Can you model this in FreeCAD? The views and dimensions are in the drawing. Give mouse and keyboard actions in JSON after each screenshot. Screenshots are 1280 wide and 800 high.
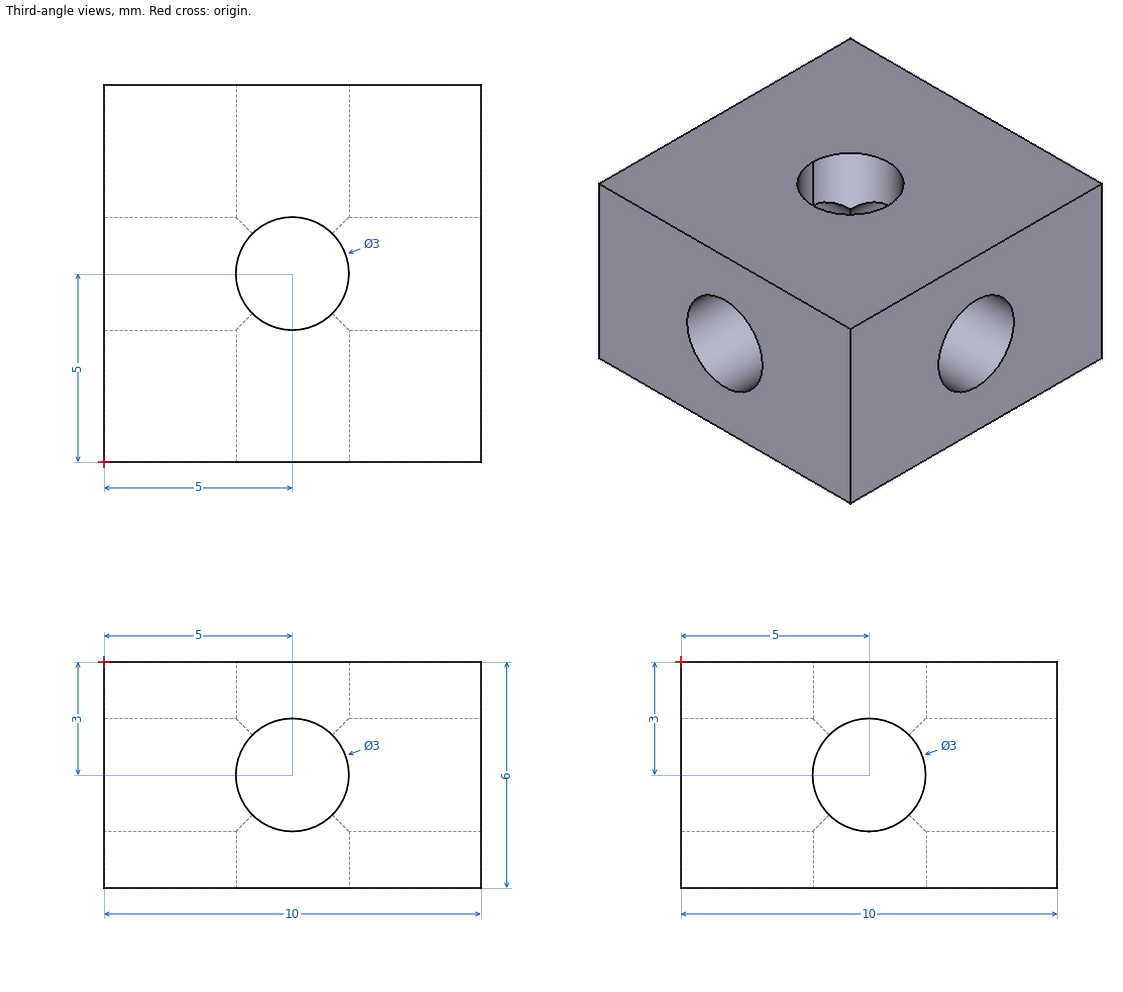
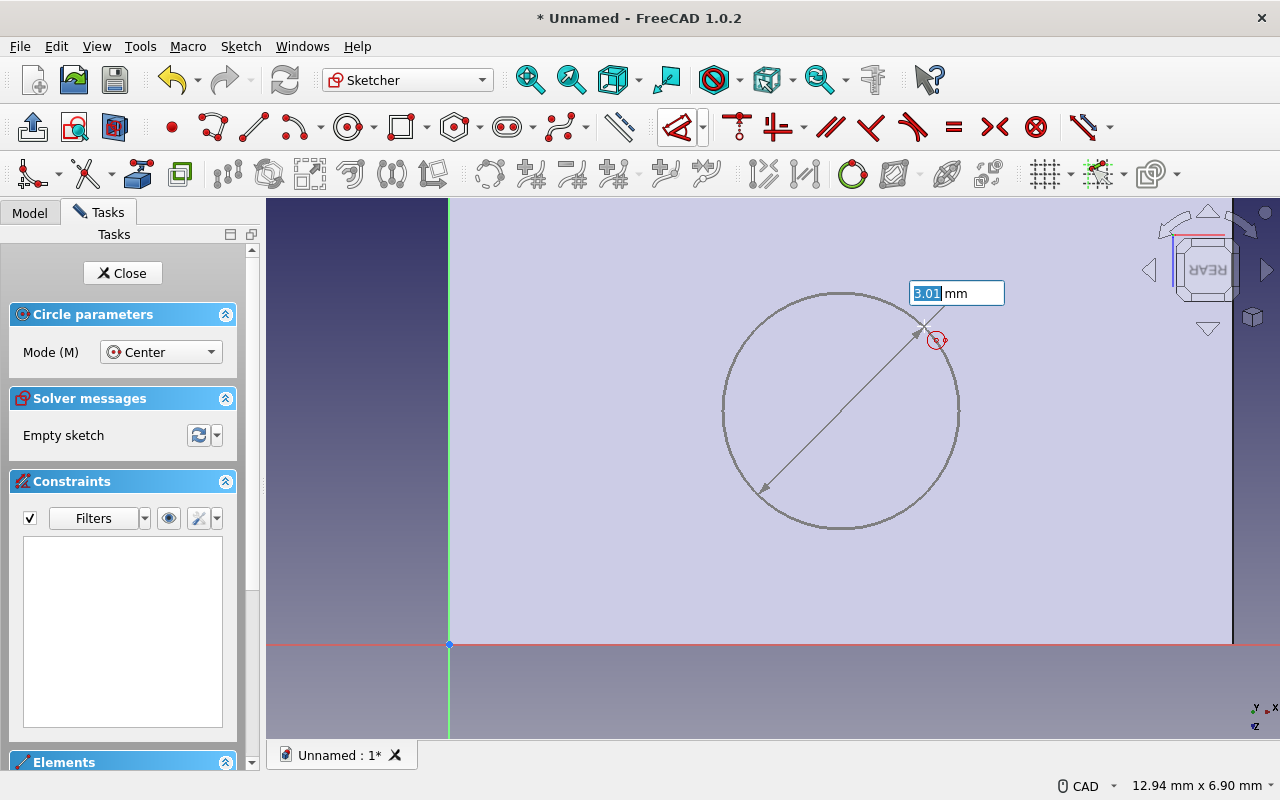
{"action": "type", "text": "3"}
{"action": "key", "text": "Return"}
{"action": "key", "text": "Escape"}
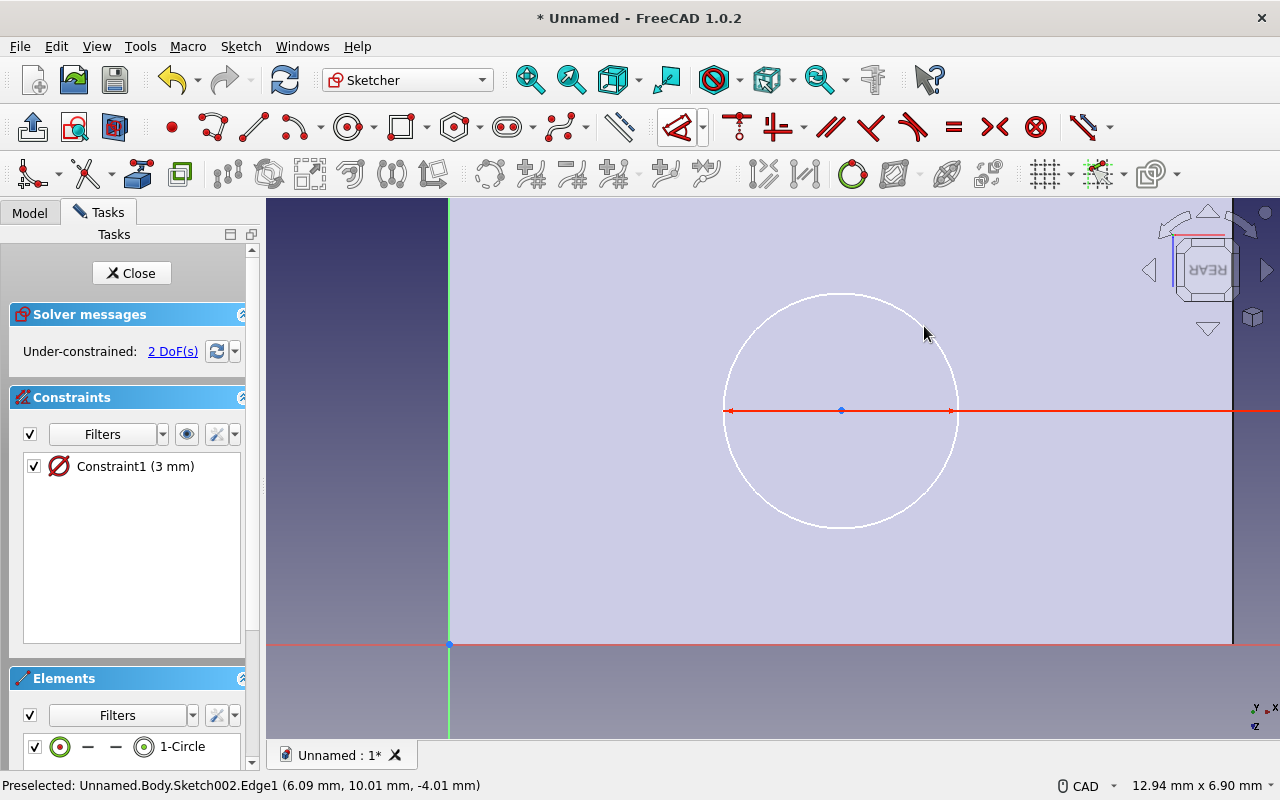
{"action": "left_click", "coordinate": [841, 411]}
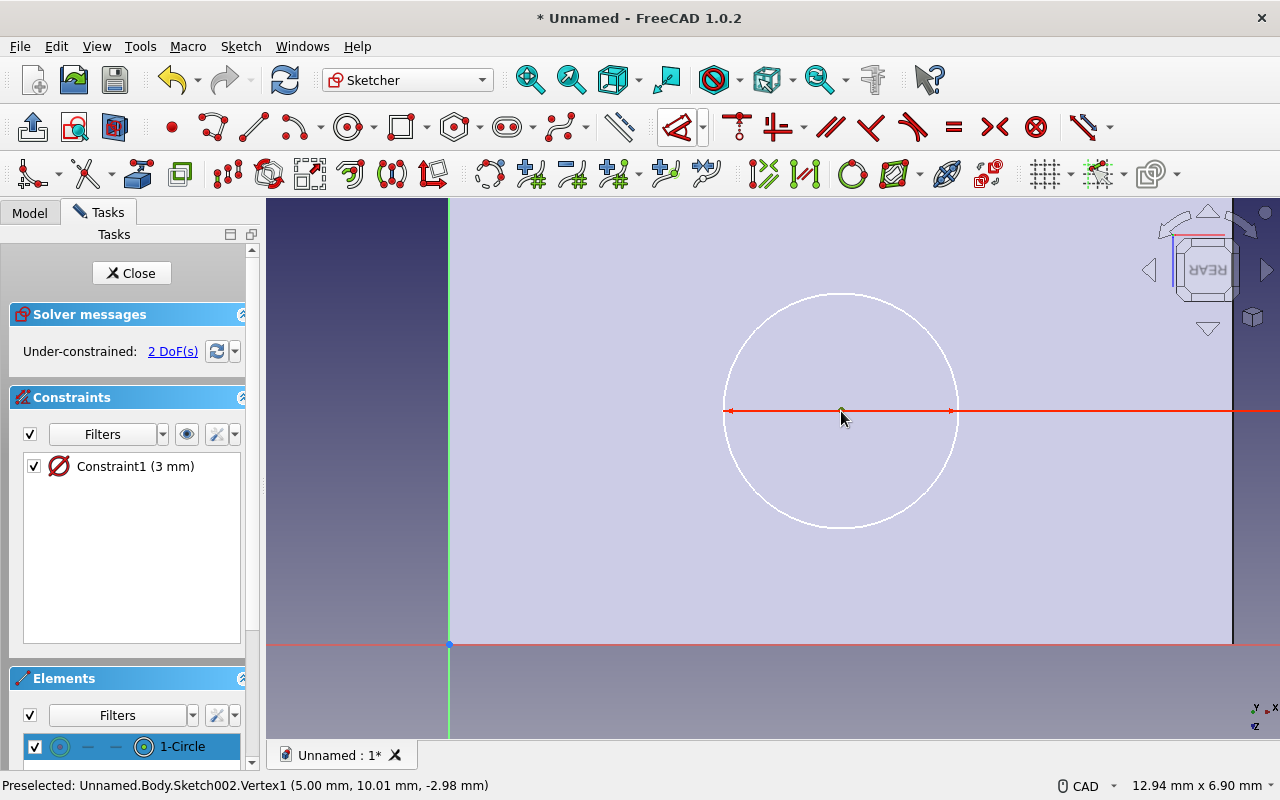
{"action": "key", "text": "l"}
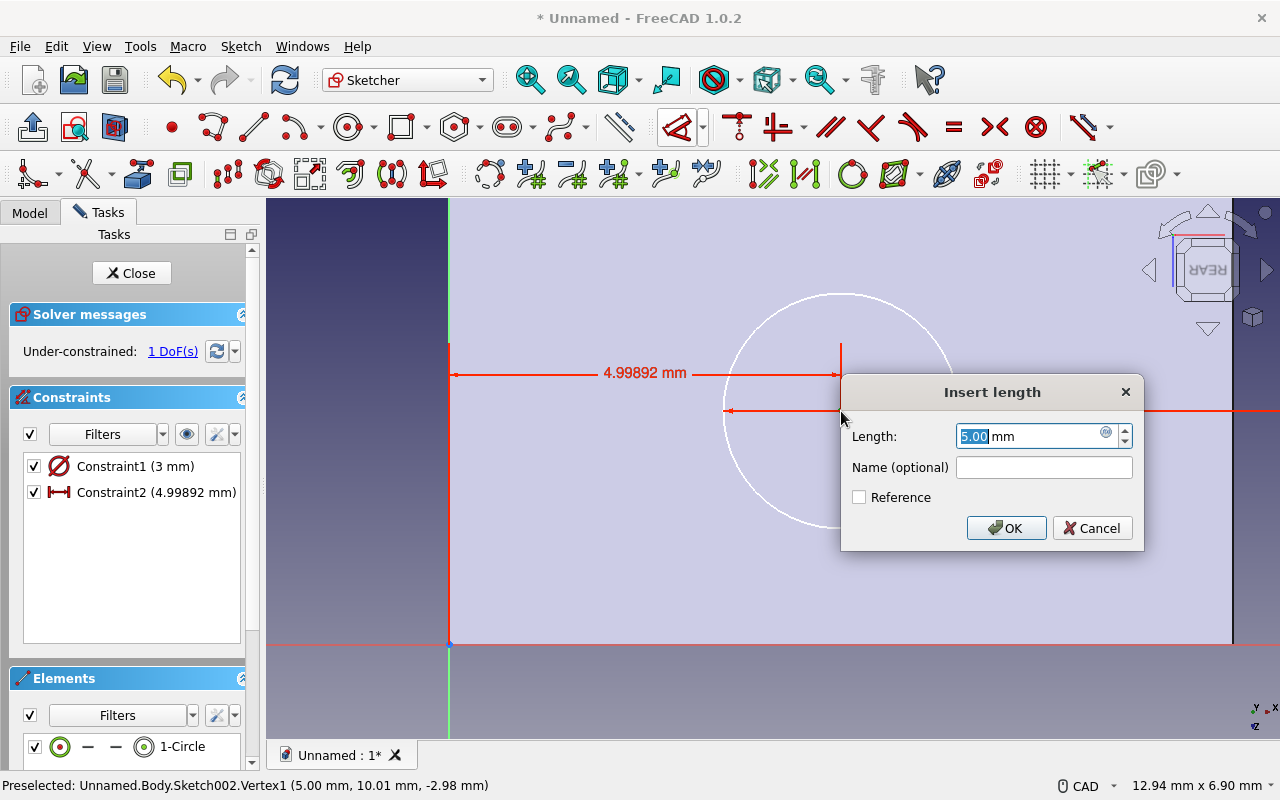
{"action": "type", "text": "5"}
{"action": "key", "text": "Return"}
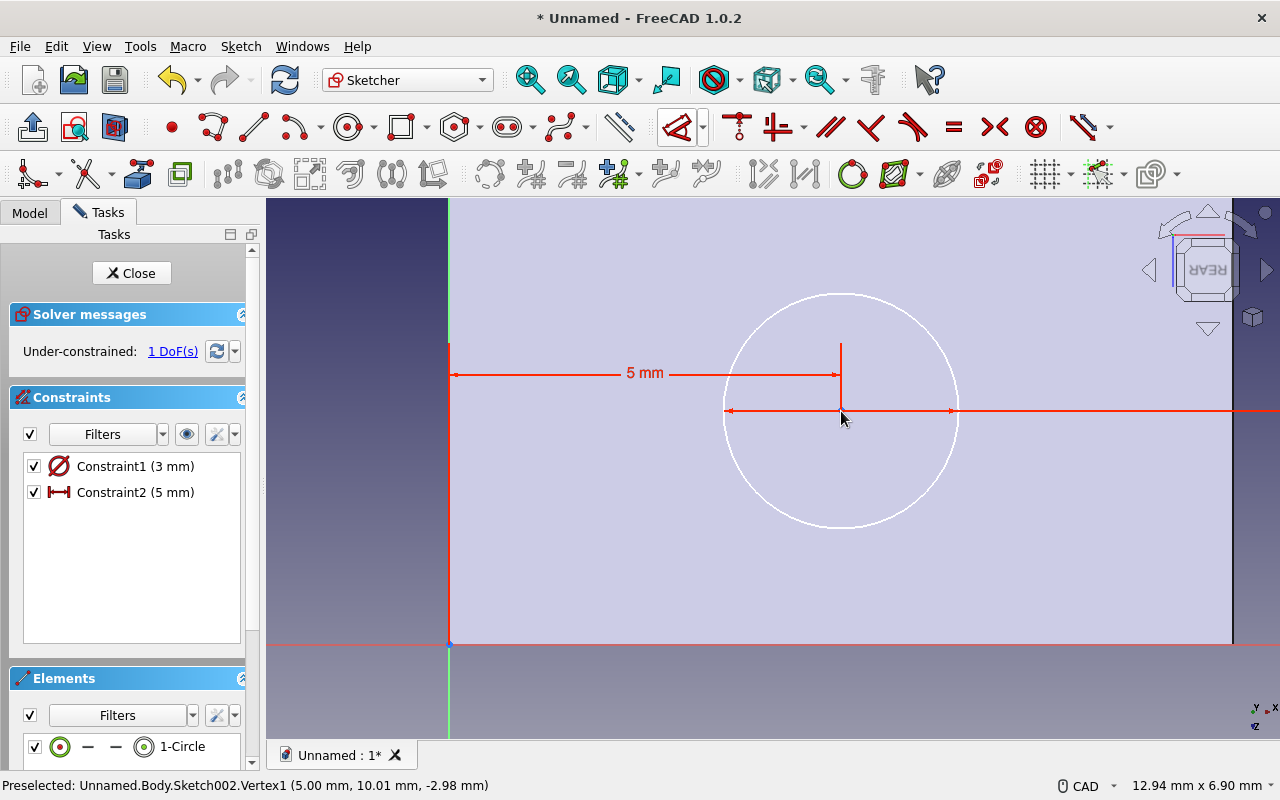
{"action": "left_click", "coordinate": [841, 411]}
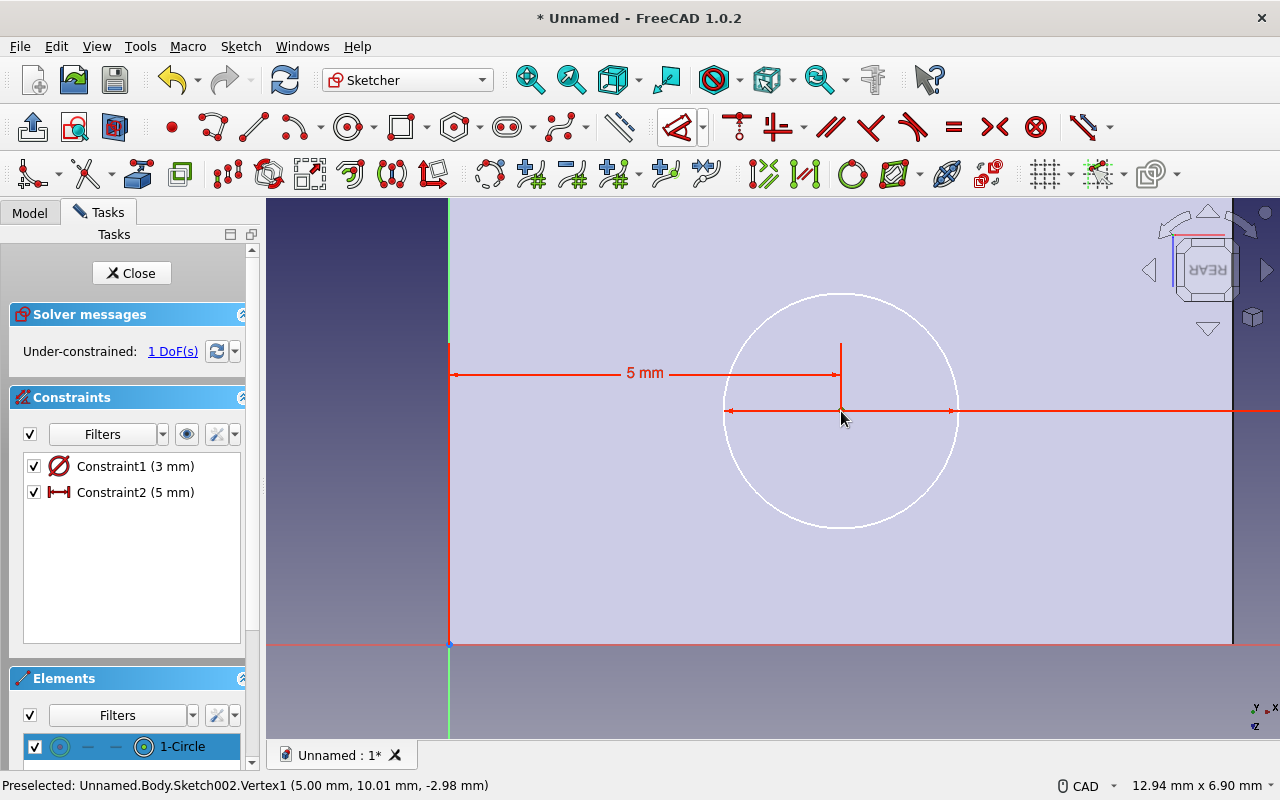
{"action": "left_click", "coordinate": [702, 128]}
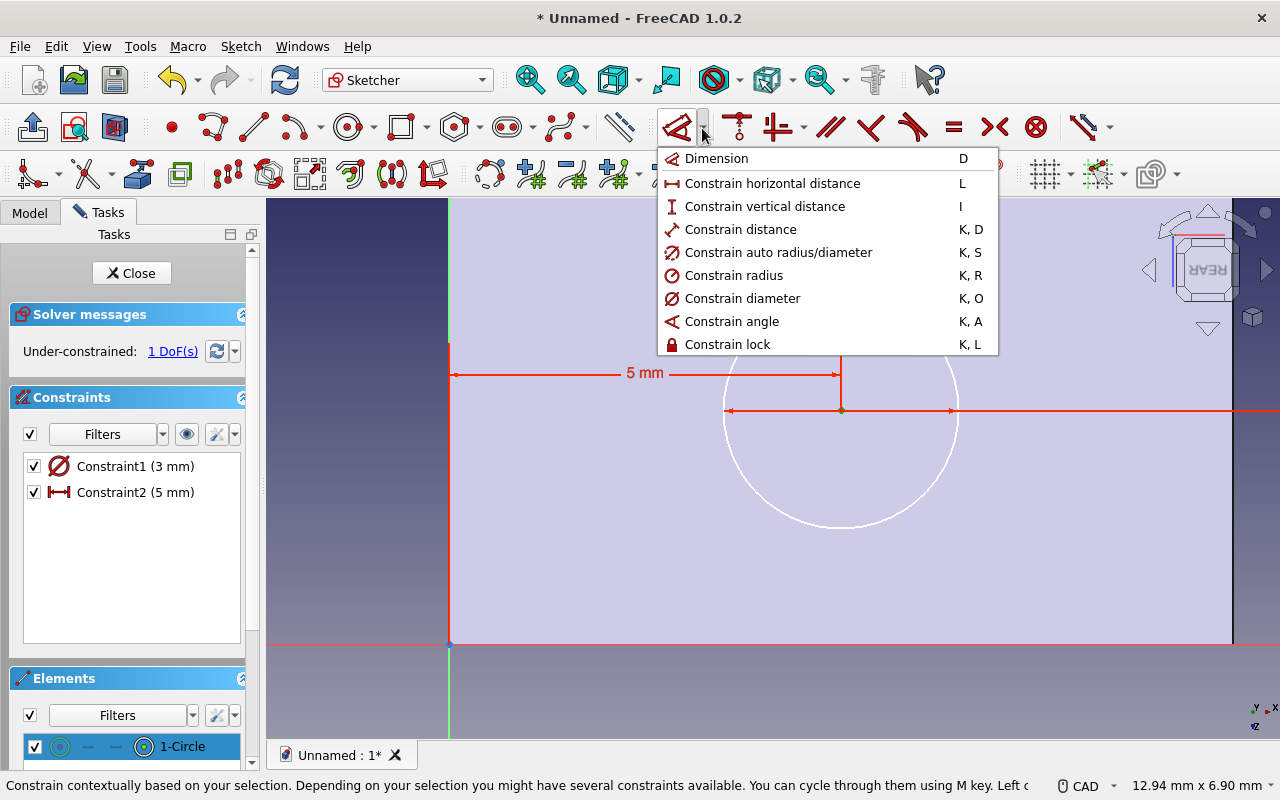
{"action": "left_click", "coordinate": [828, 206]}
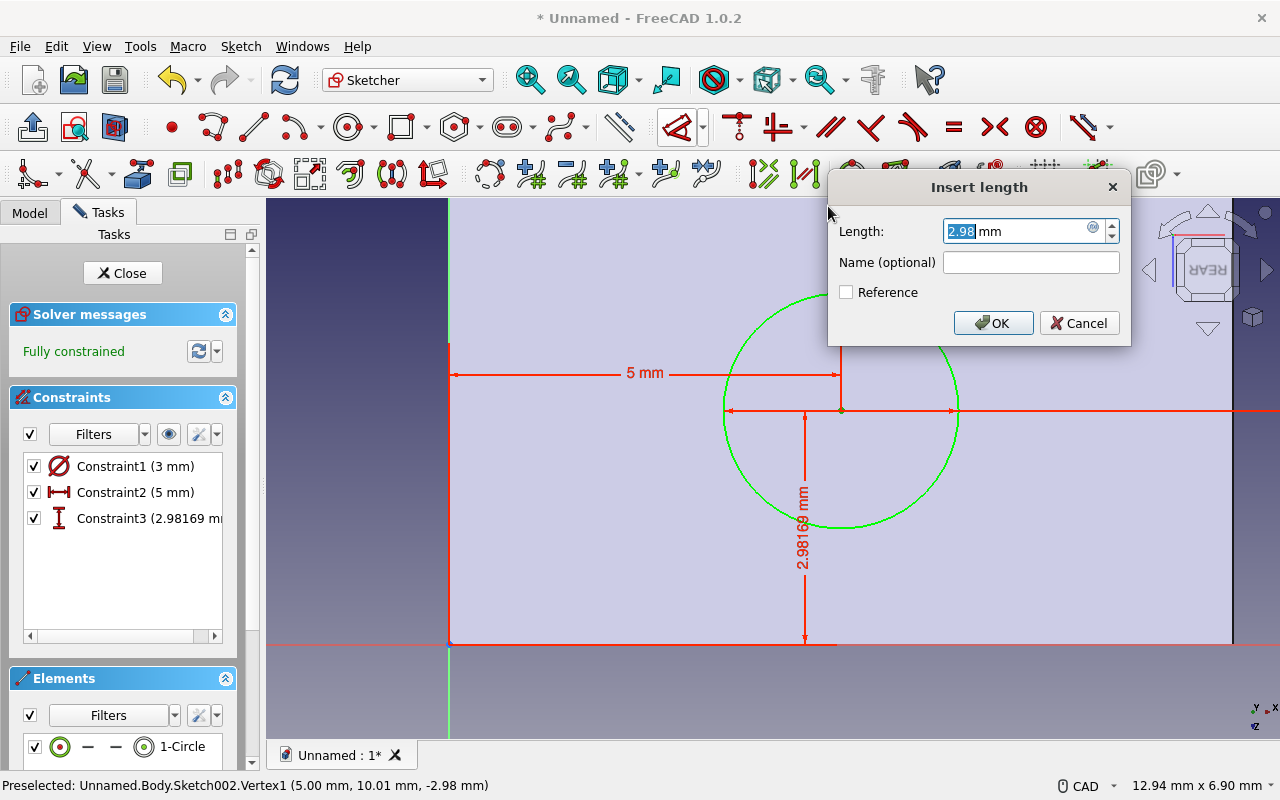
{"action": "type", "text": "3"}
{"action": "key", "text": "Return"}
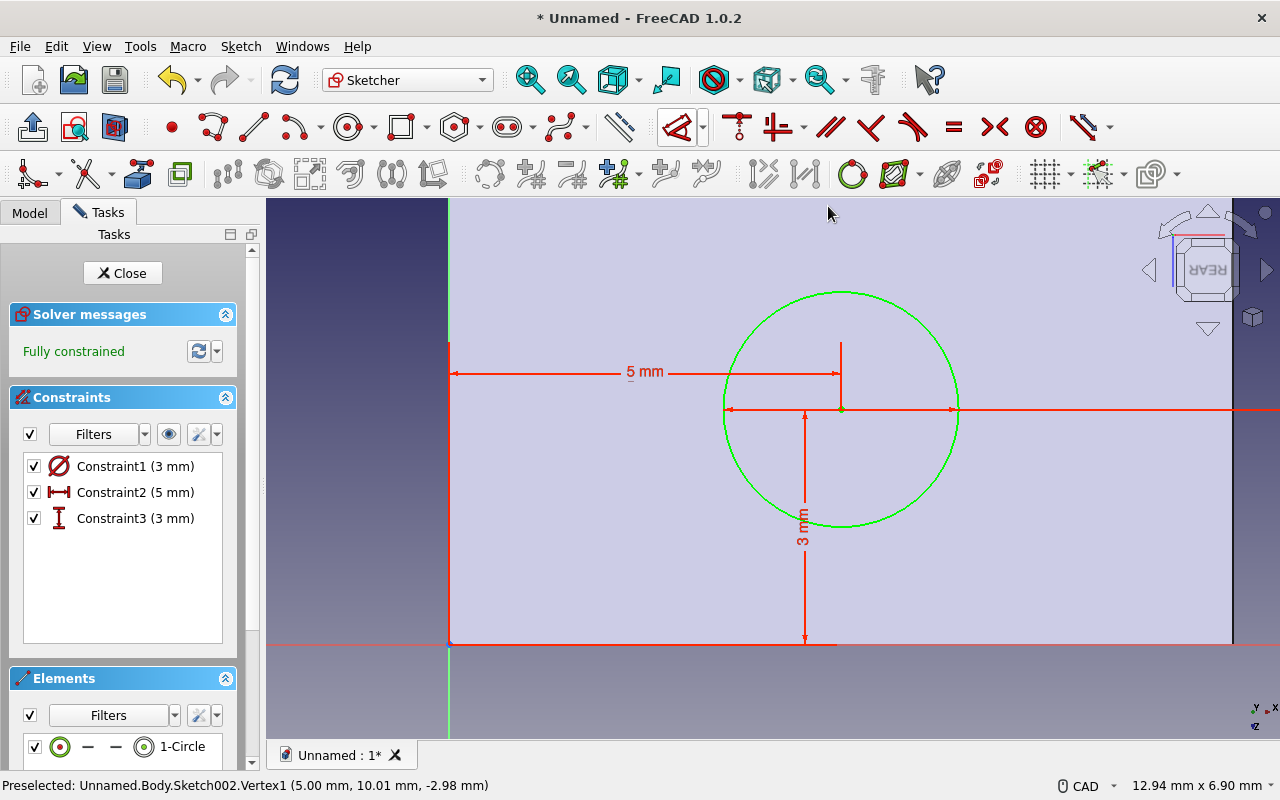
{"action": "left_click", "coordinate": [123, 273]}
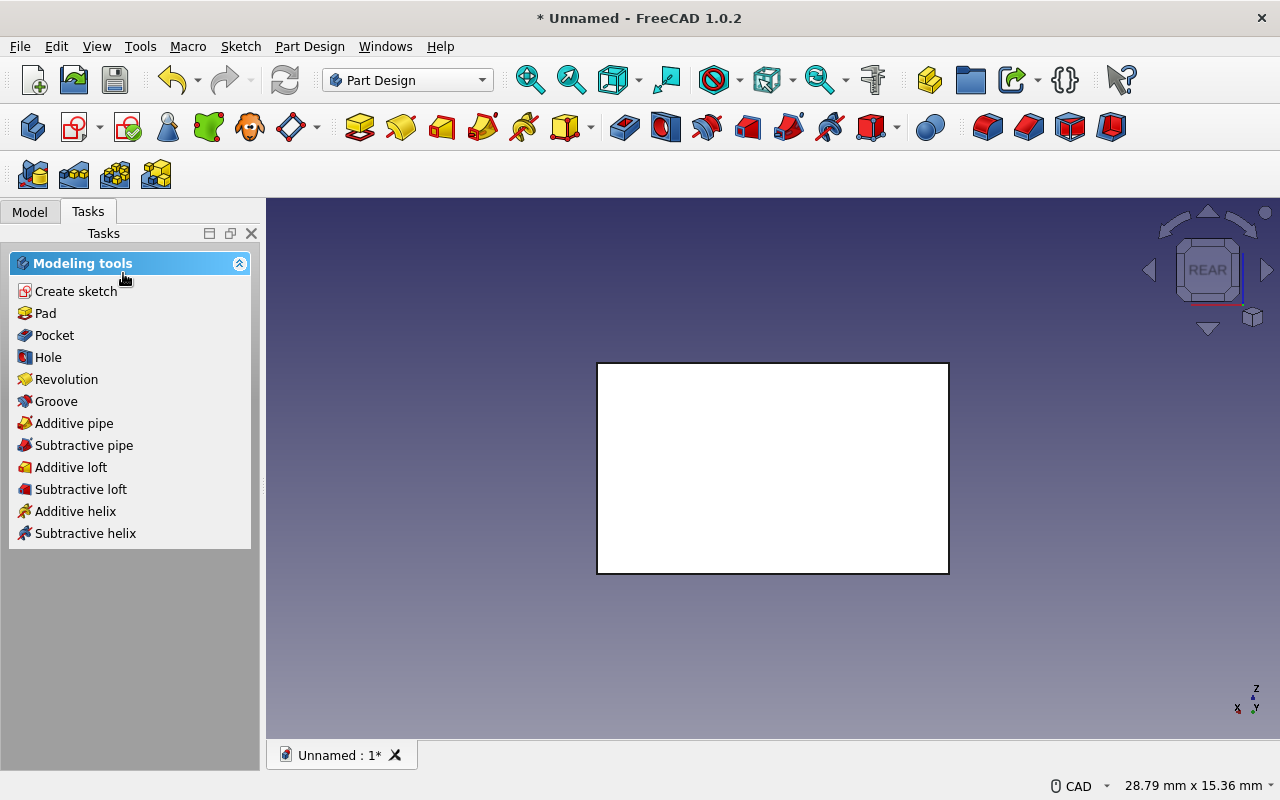
{"action": "left_click", "coordinate": [625, 128]}